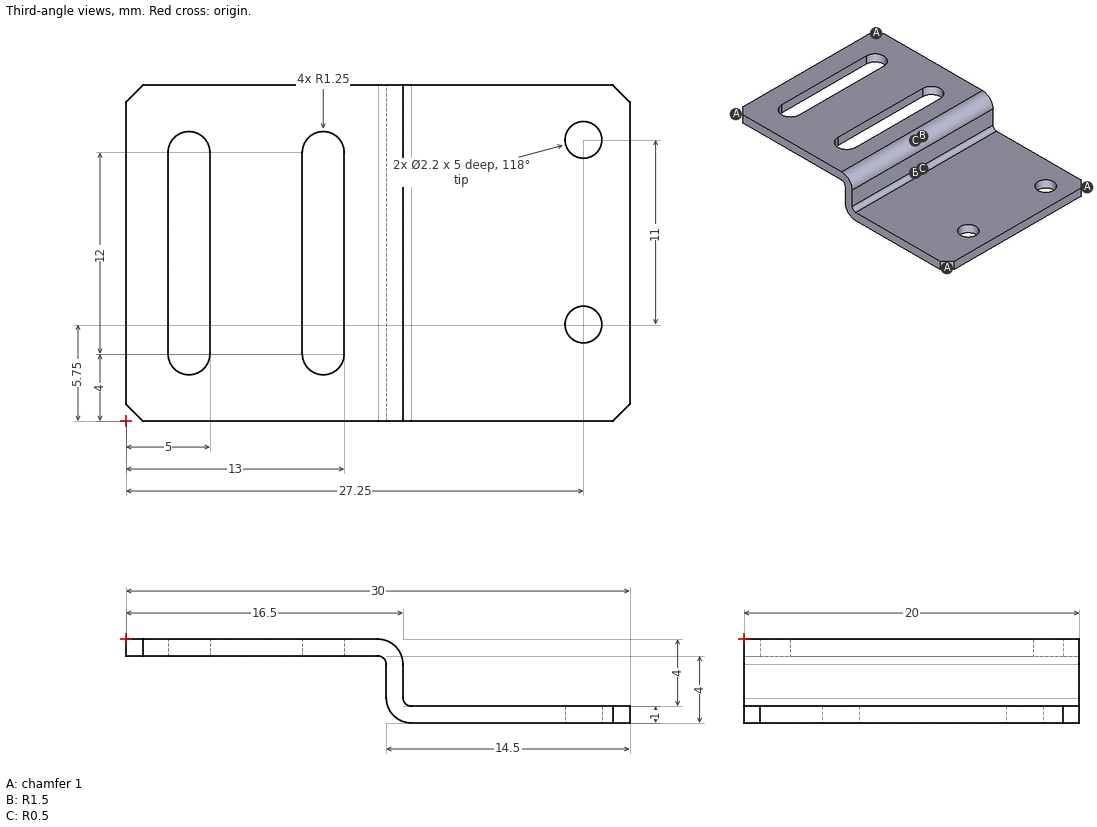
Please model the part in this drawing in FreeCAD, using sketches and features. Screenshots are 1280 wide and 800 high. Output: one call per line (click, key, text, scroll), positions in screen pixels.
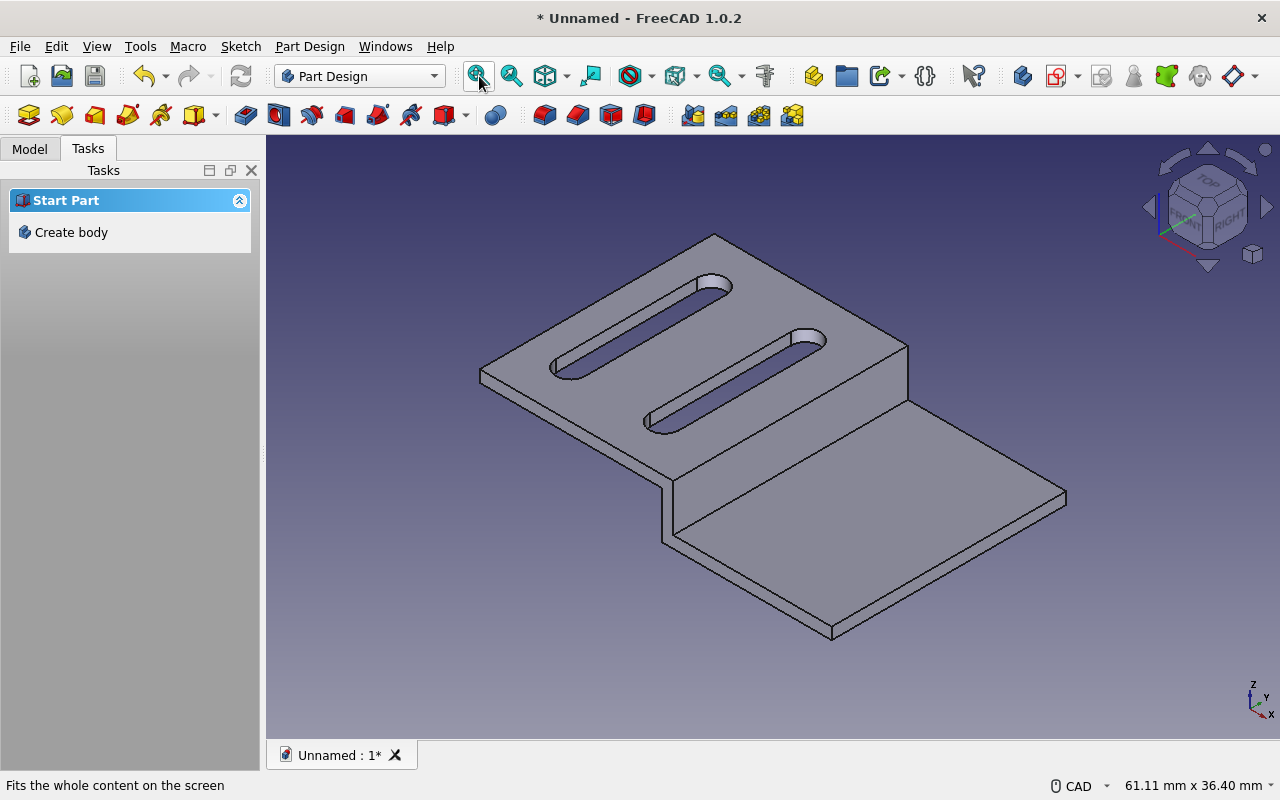
click(832, 632)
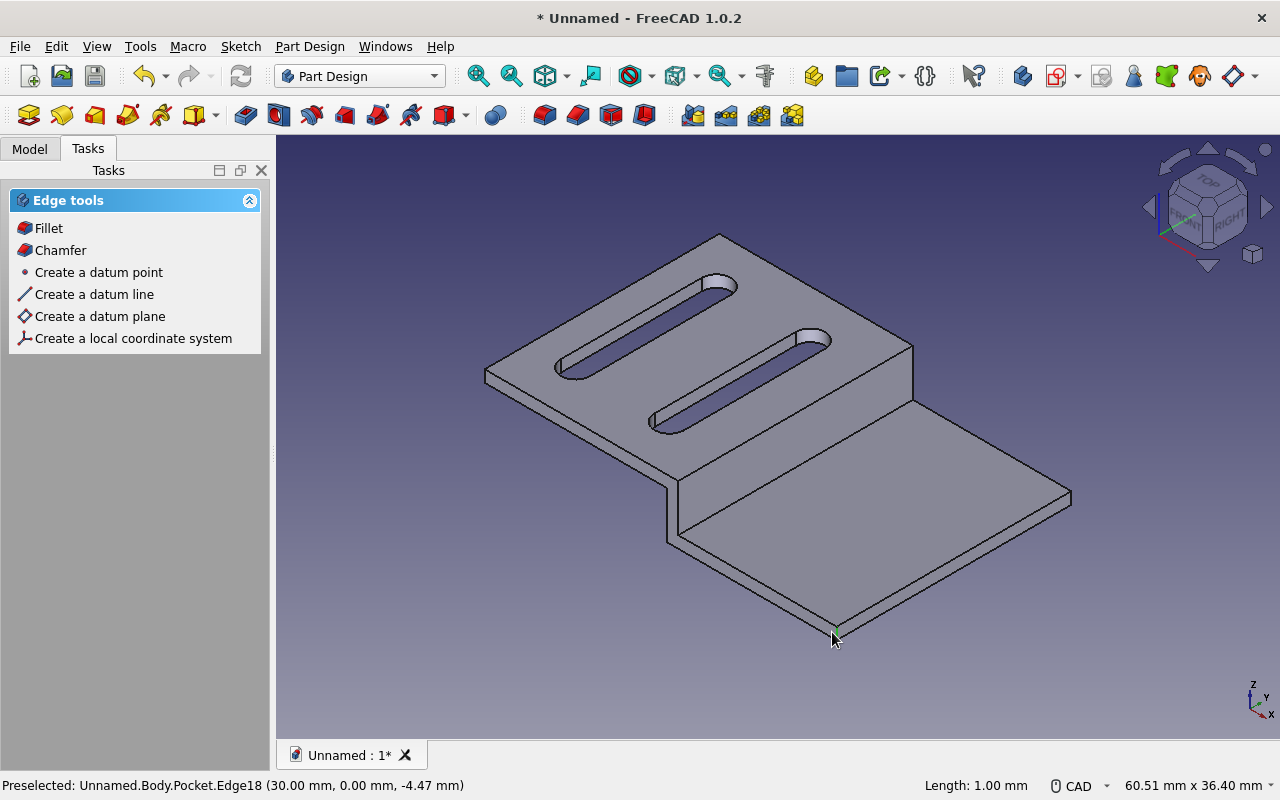
scroll(485, 375, up, 5)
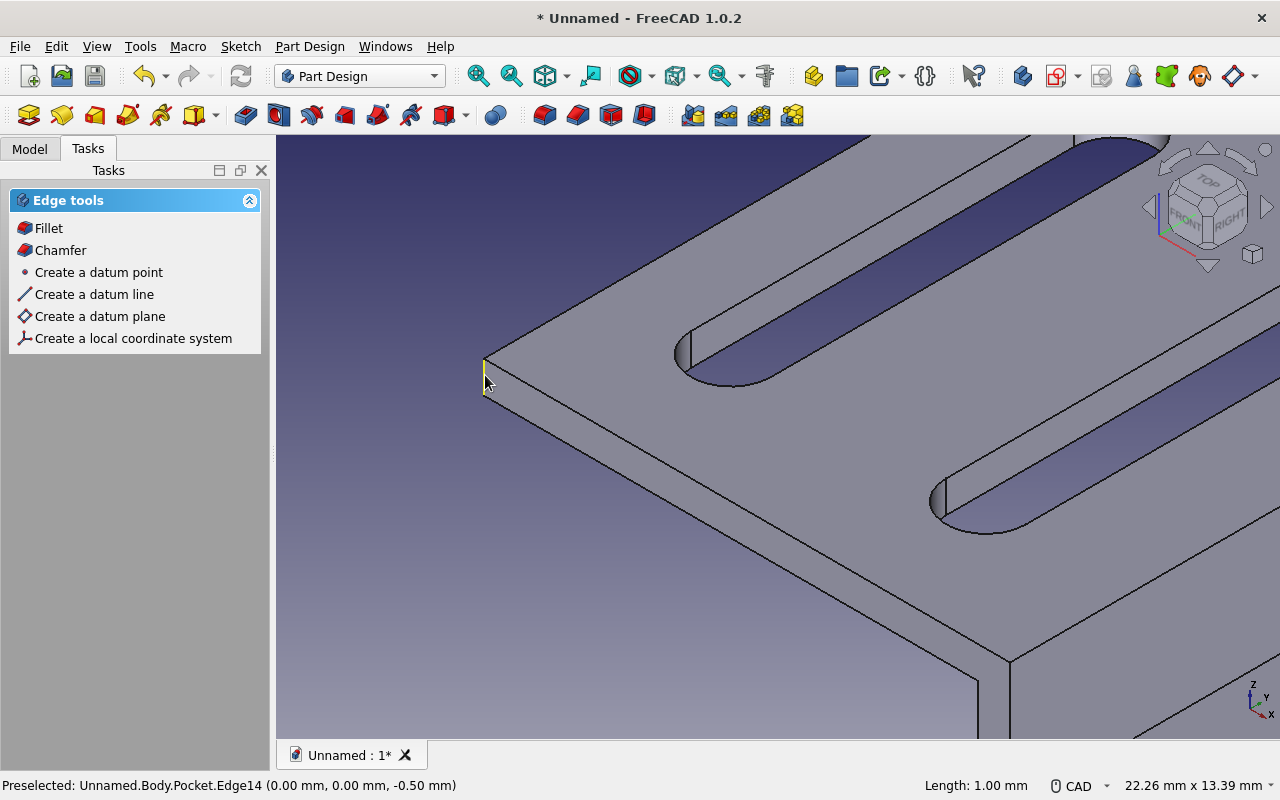
click(479, 76)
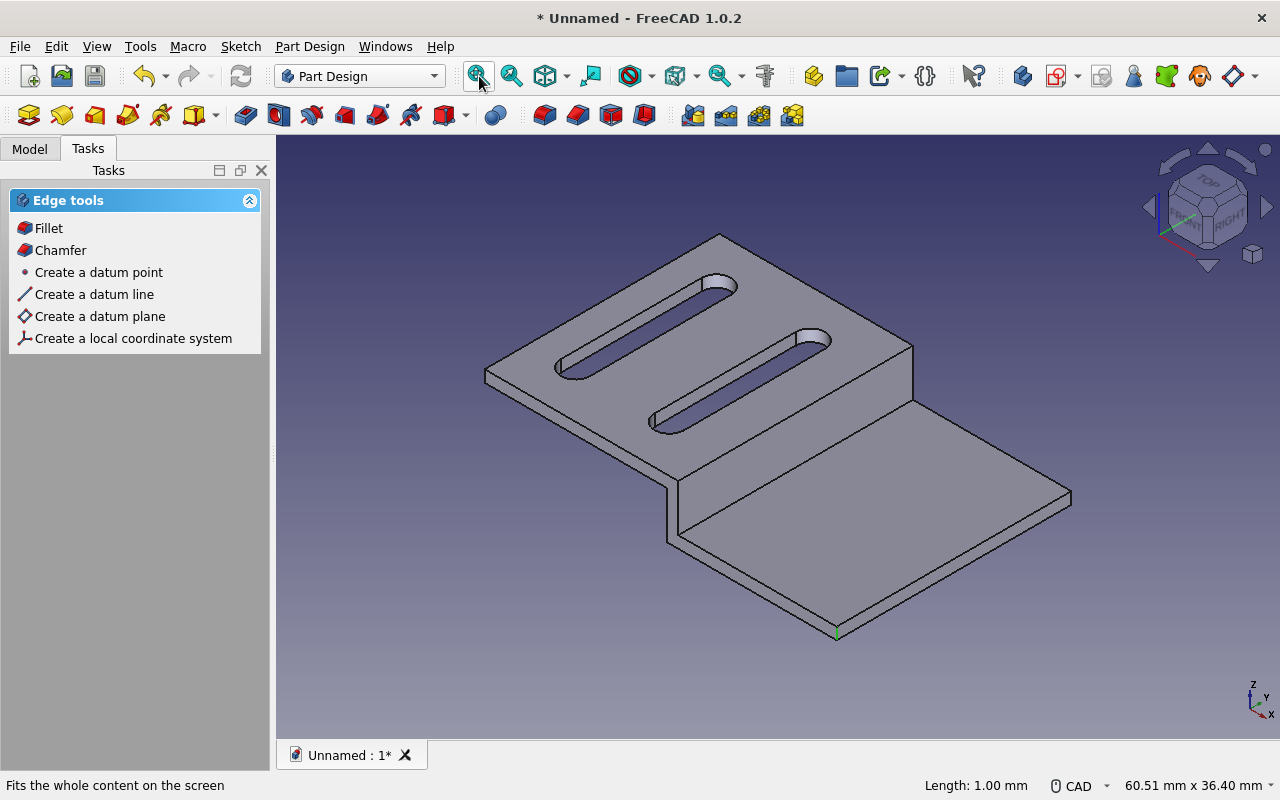
key(2)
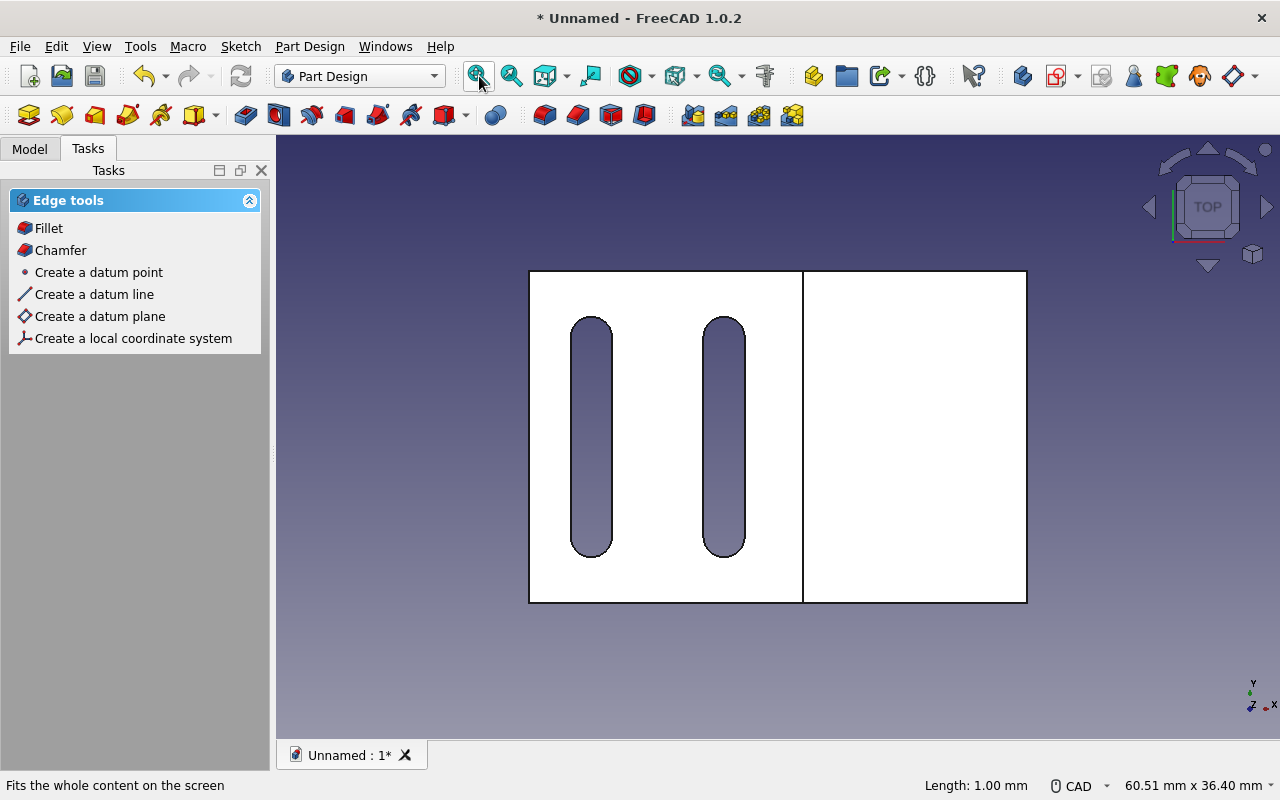
scroll(529, 602, up, 5)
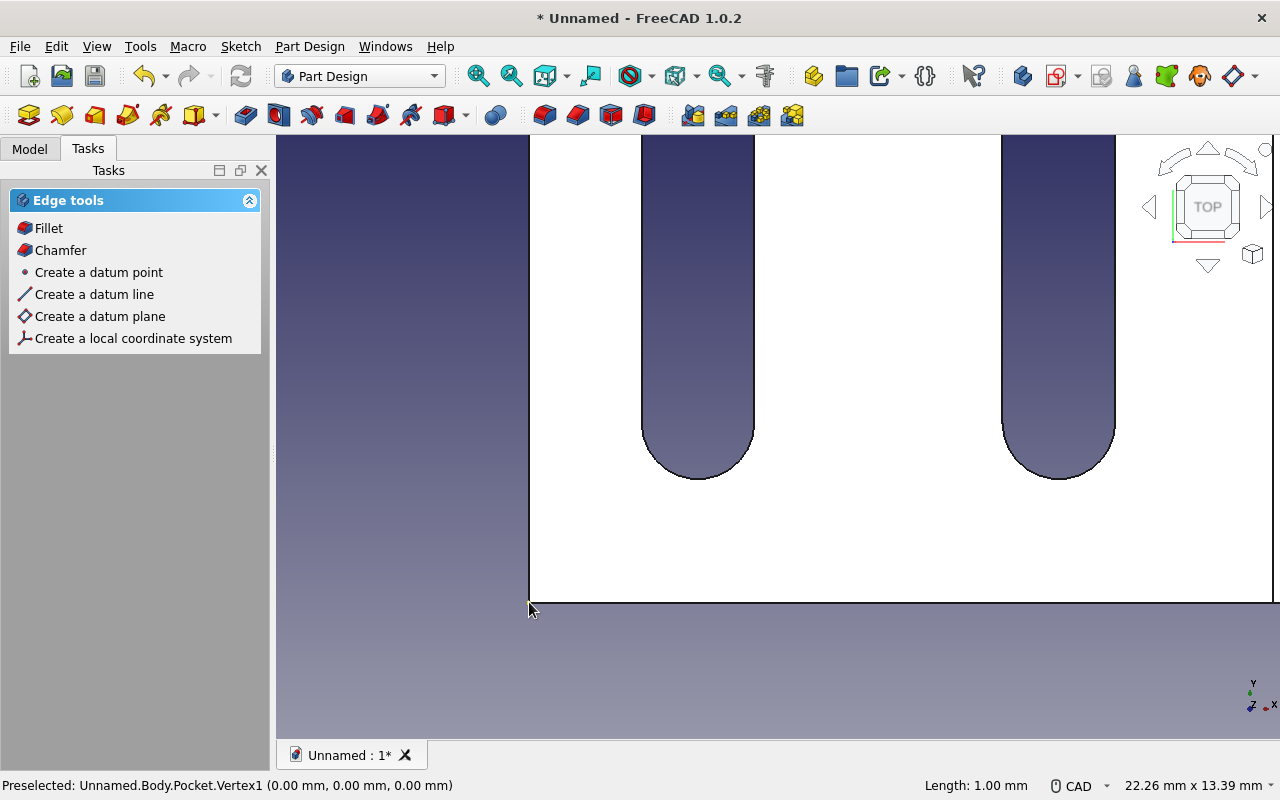
click(479, 76)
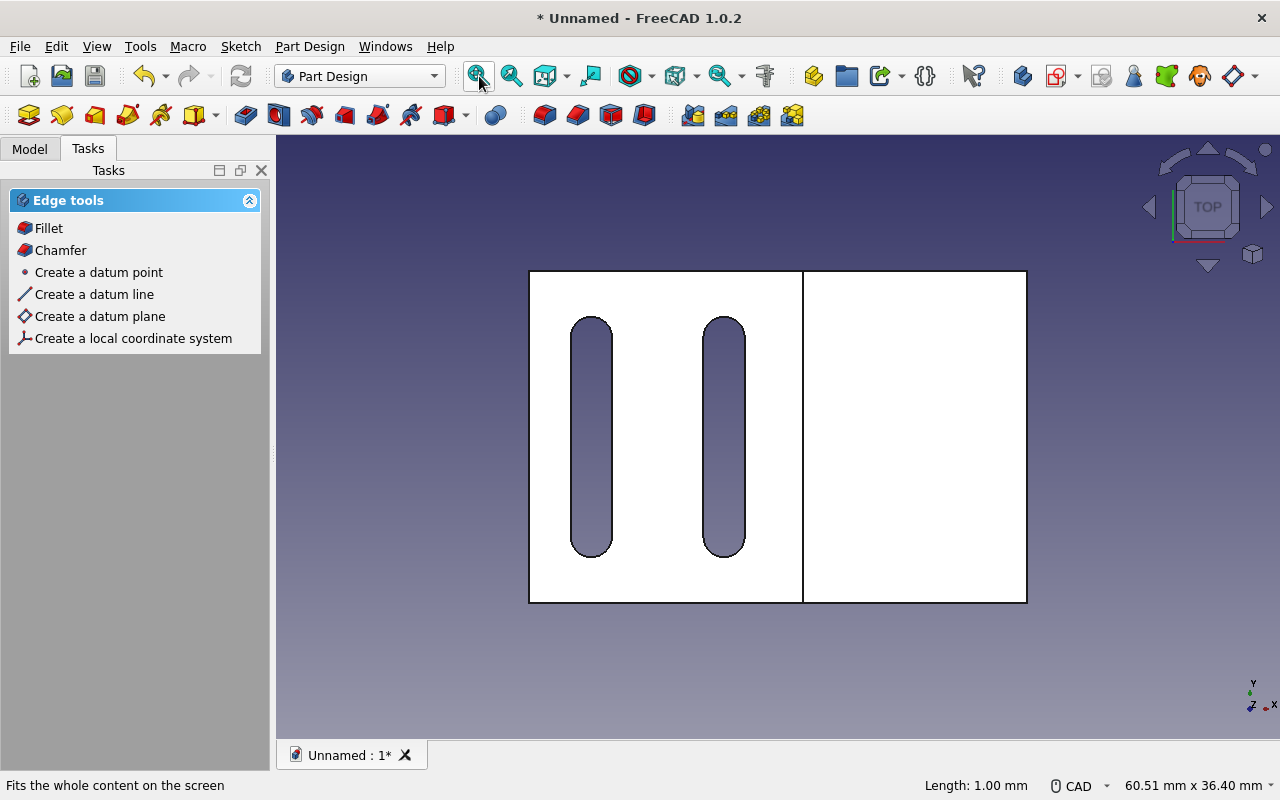
key(1)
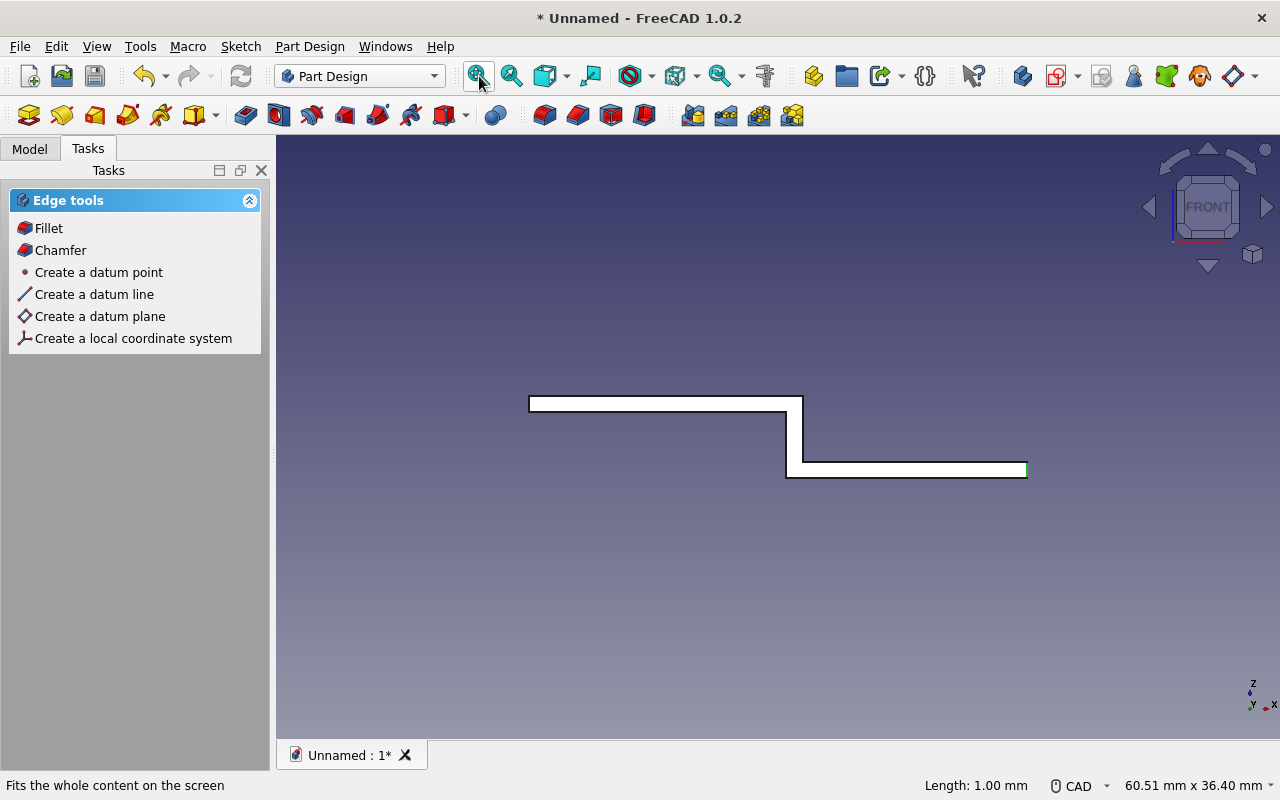
scroll(529, 403, up, 5)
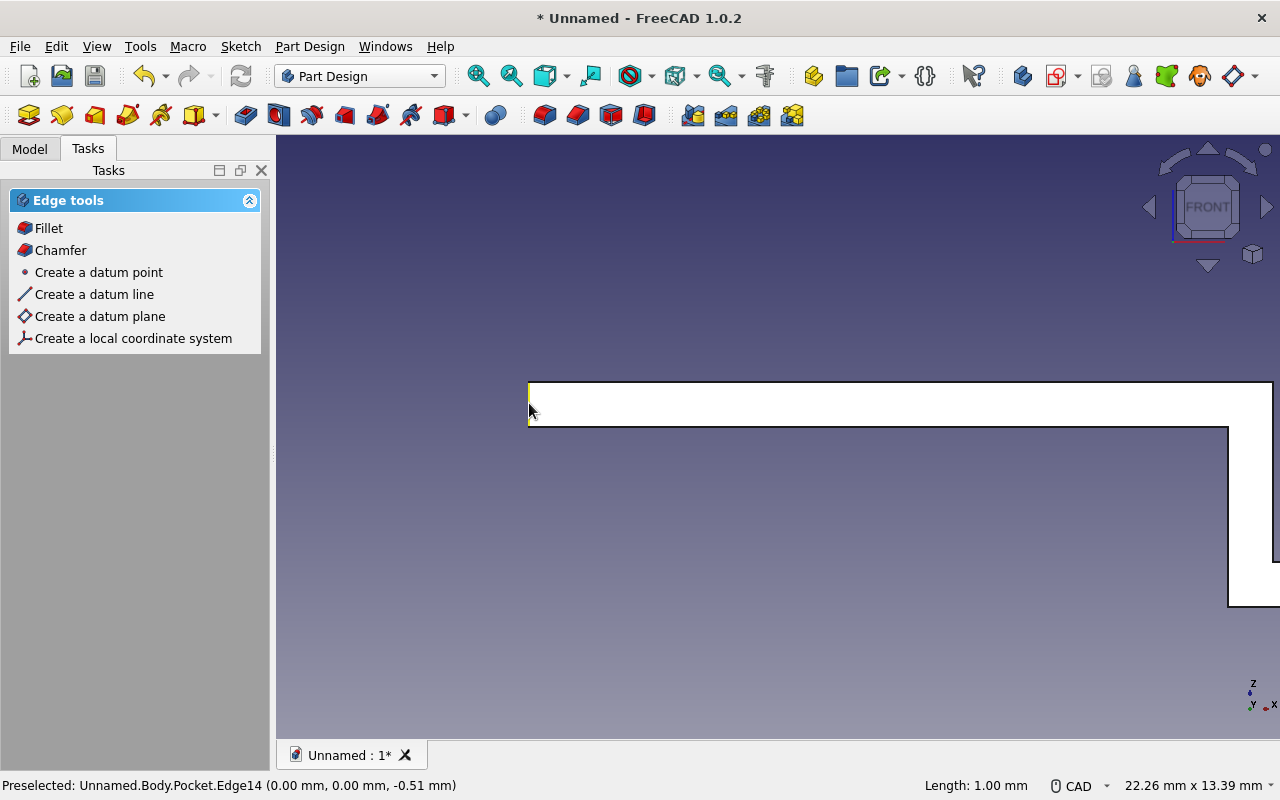
click(479, 76)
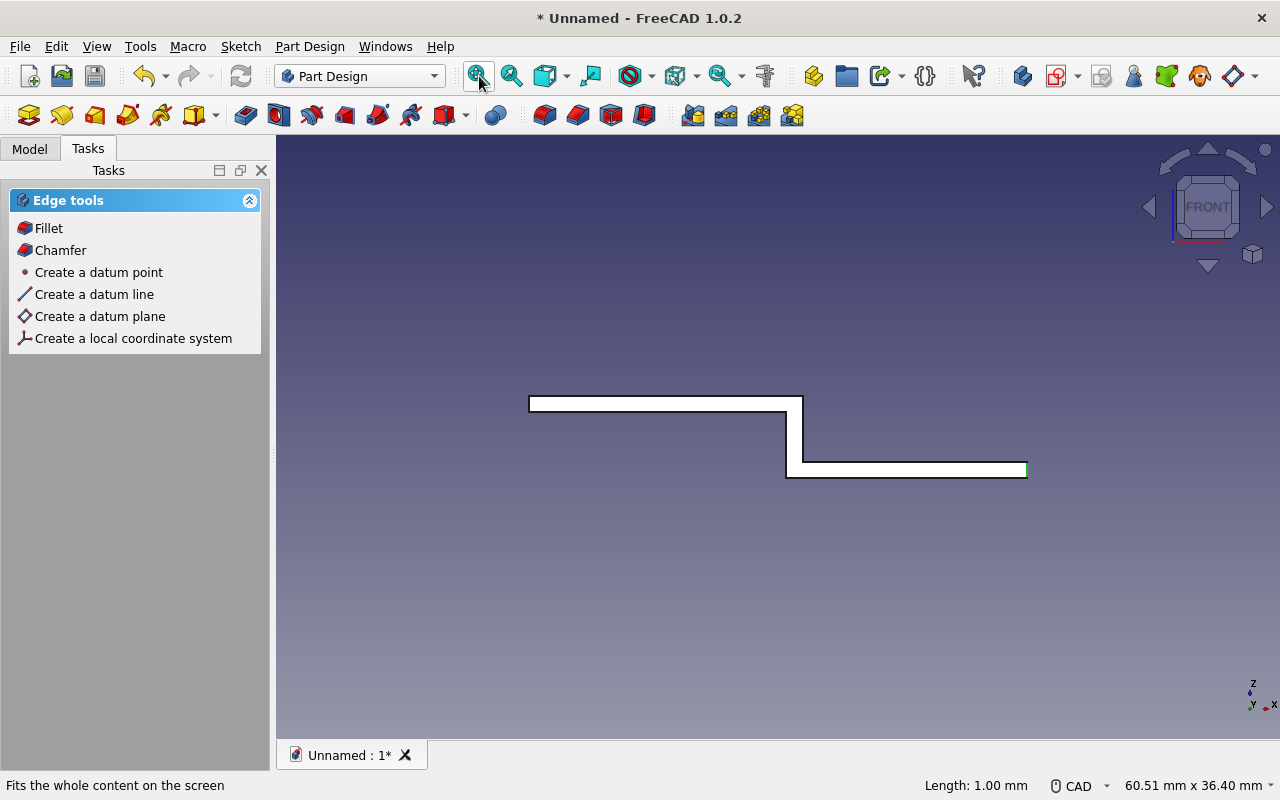
key(3)